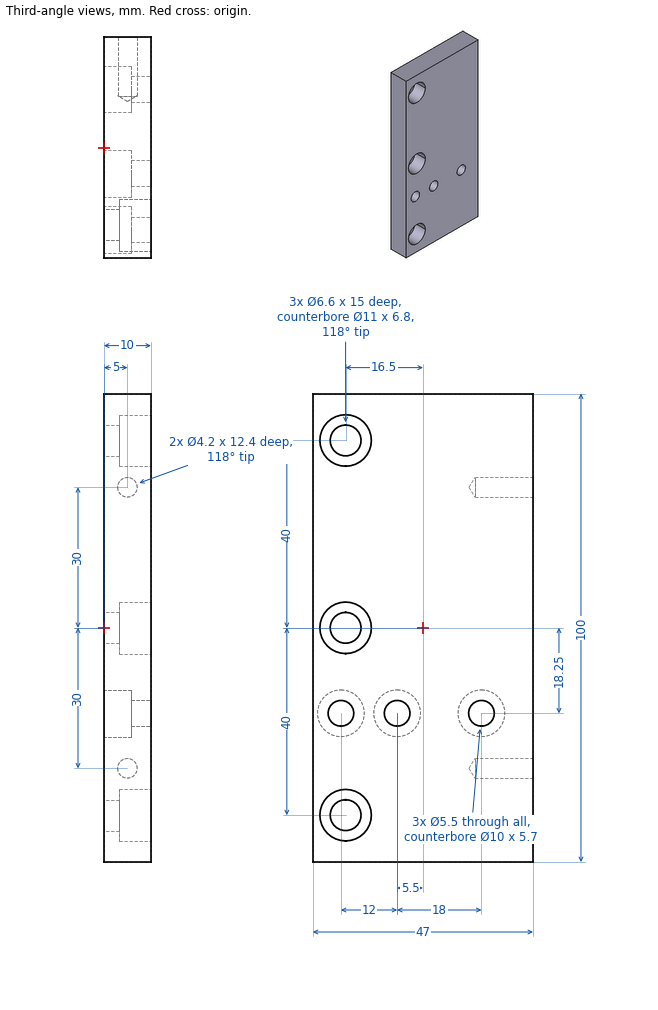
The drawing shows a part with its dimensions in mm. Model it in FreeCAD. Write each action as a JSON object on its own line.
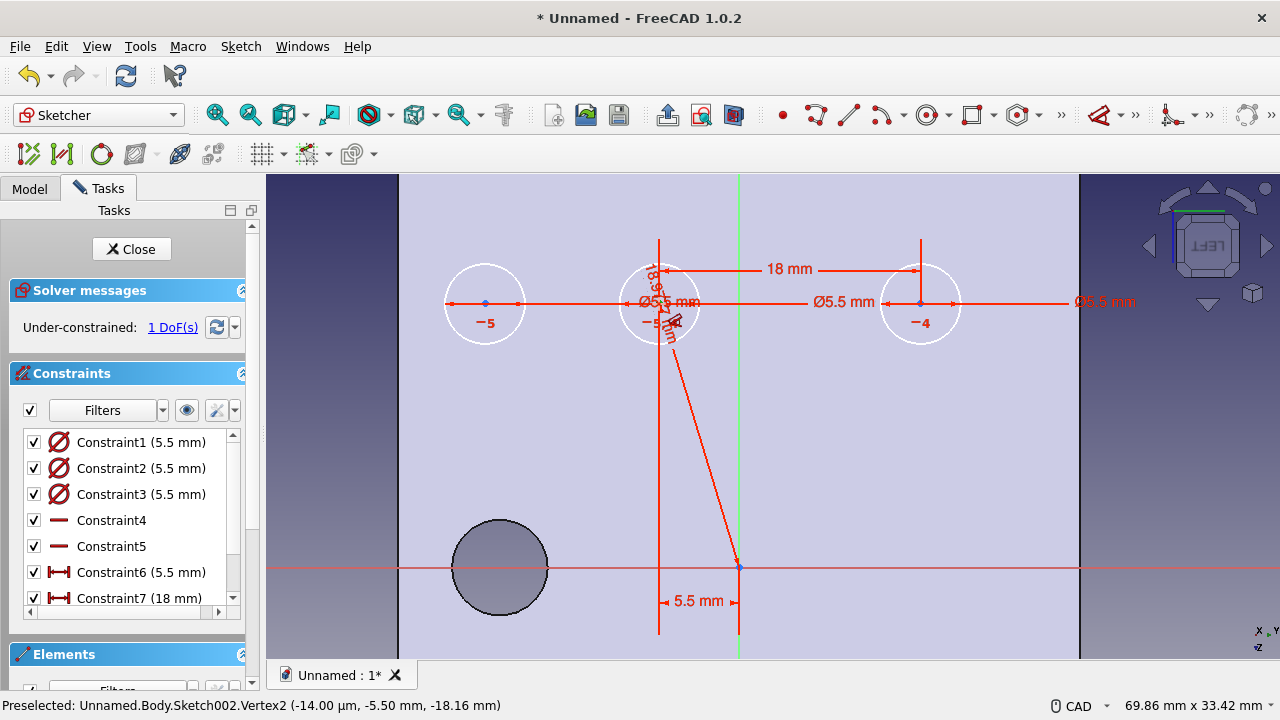
{"action": "left_click", "coordinate": [485, 304]}
{"action": "left_click", "coordinate": [572, 270]}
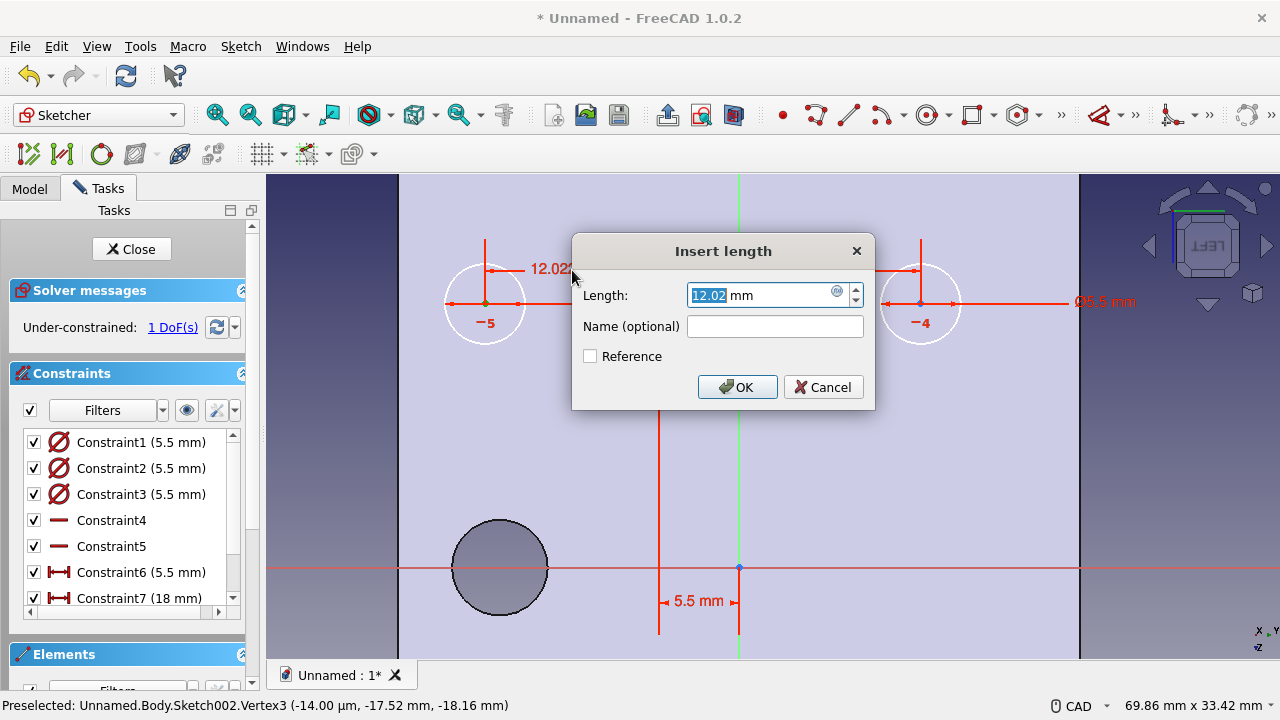
{"action": "type", "text": "12"}
{"action": "key", "text": "Return"}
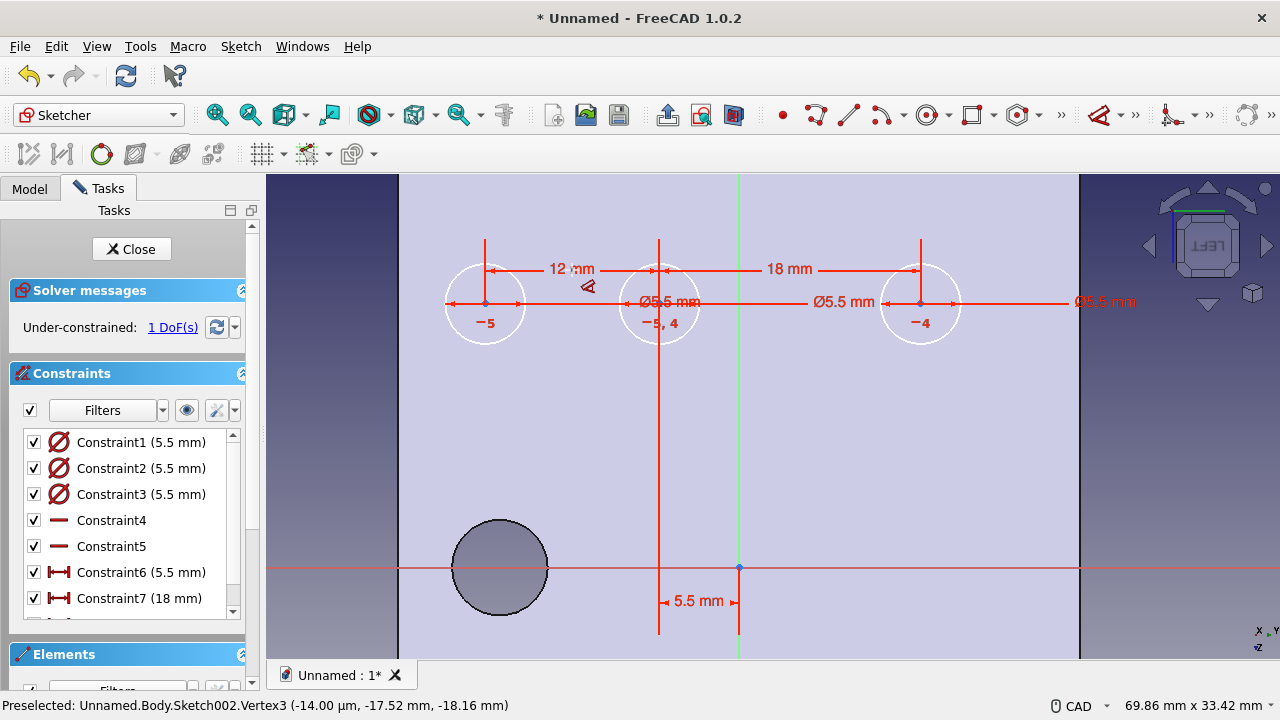
{"action": "left_click", "coordinate": [921, 304]}
{"action": "left_click", "coordinate": [955, 436]}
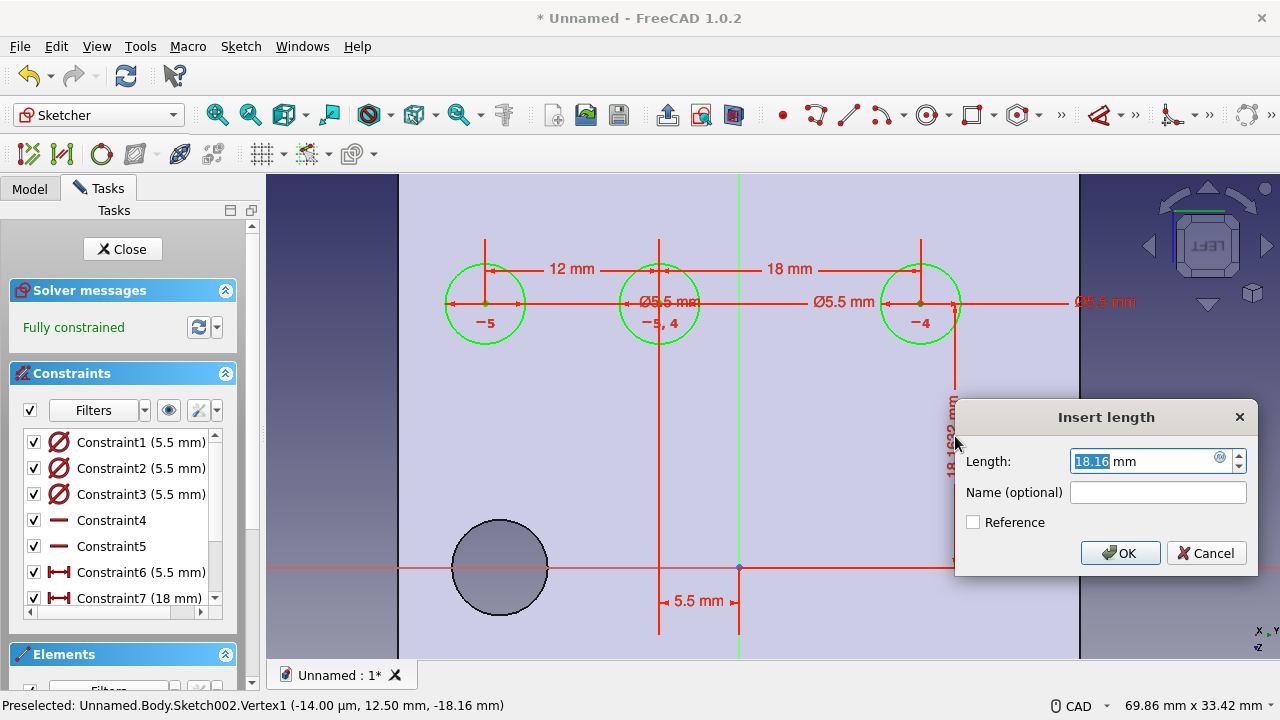
{"action": "type", "text": "18.25"}
{"action": "key", "text": "Return"}
{"action": "key", "text": "Escape"}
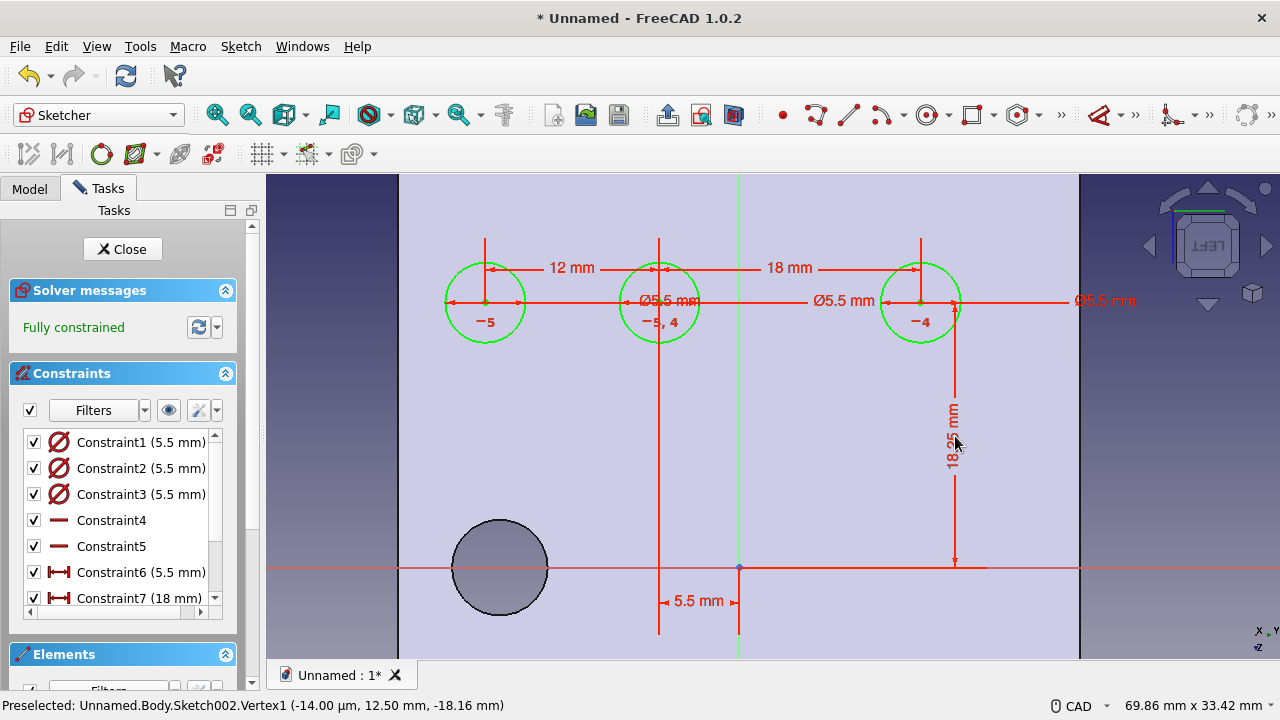
{"action": "left_click", "coordinate": [123, 249]}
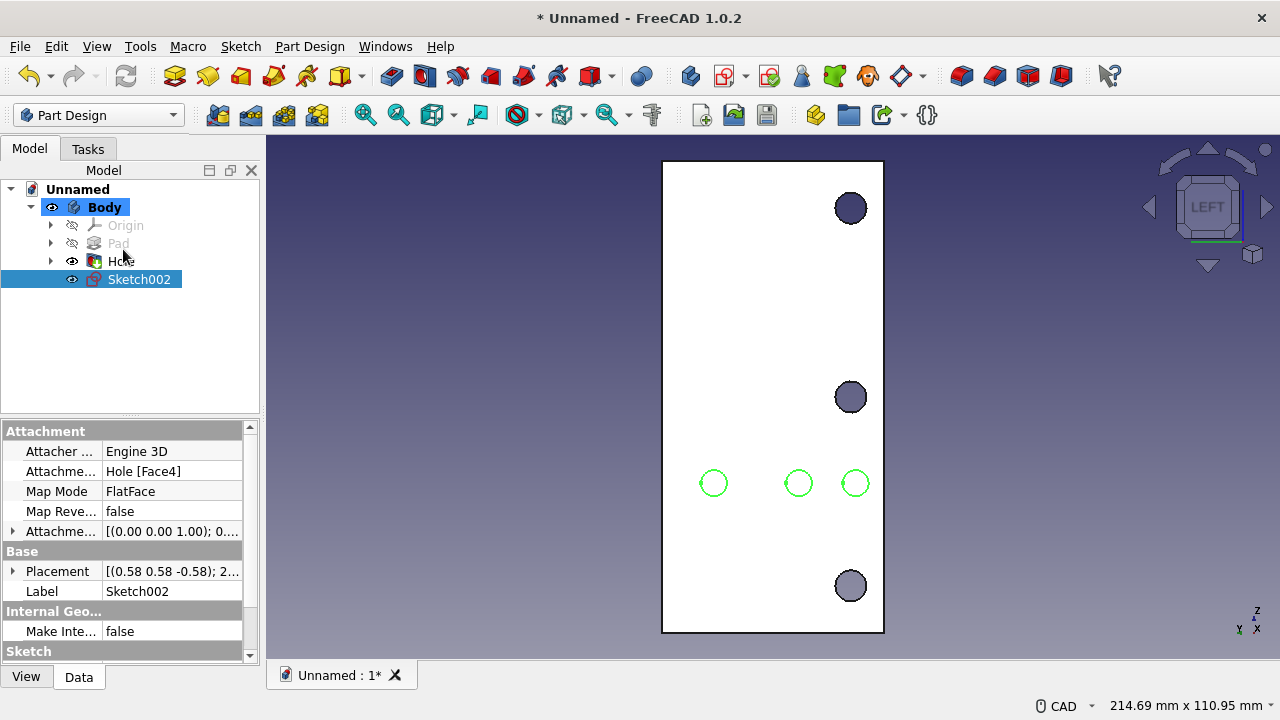
{"action": "left_click", "coordinate": [425, 76]}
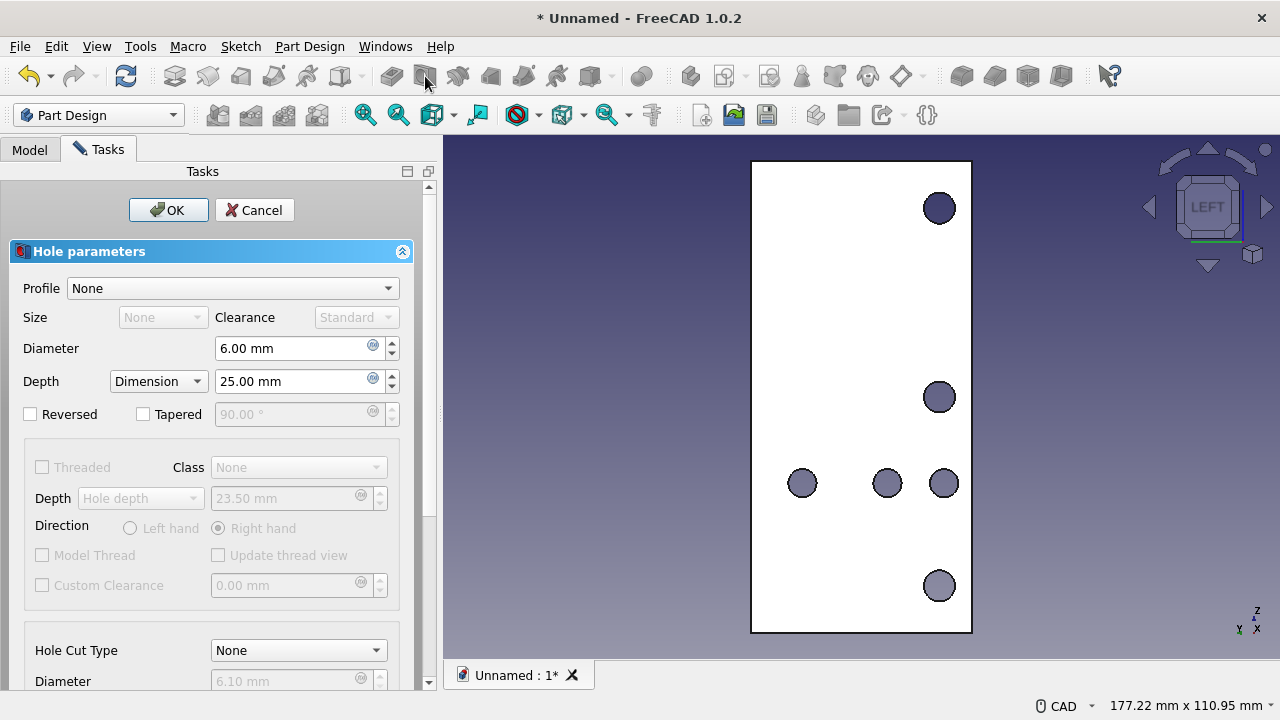
{"action": "triple_click", "coordinate": [300, 348]}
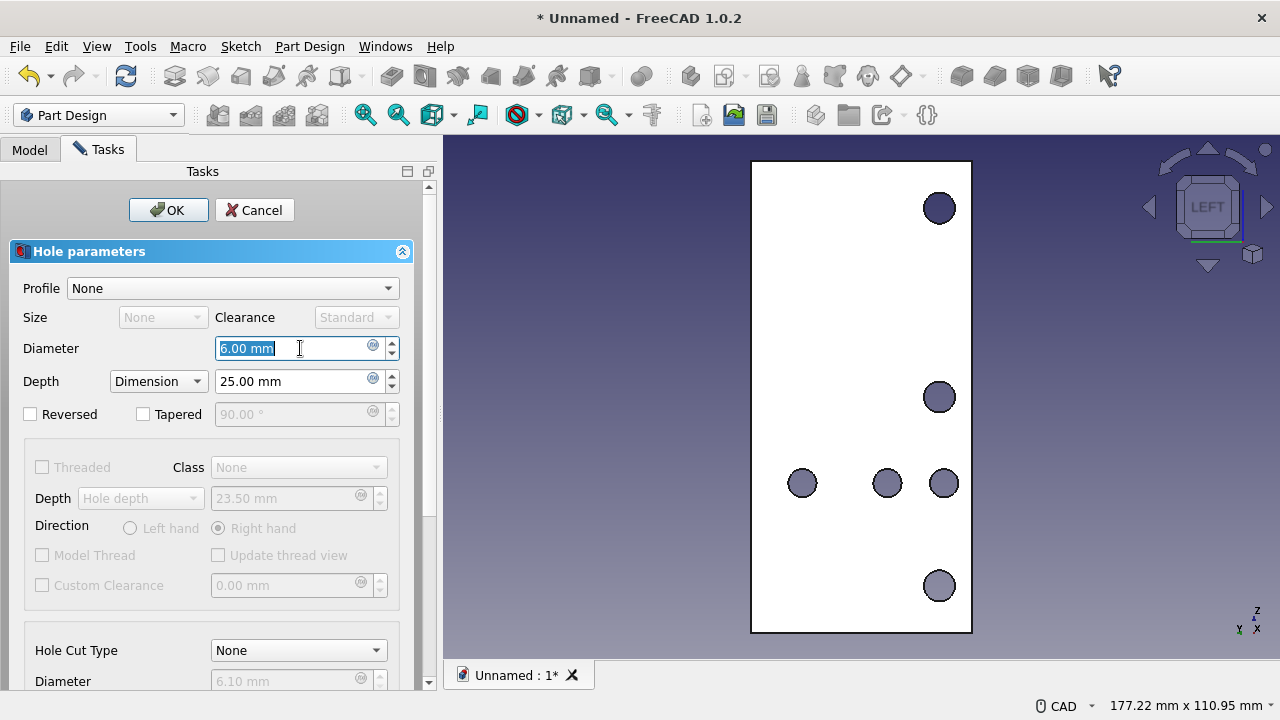
{"action": "type", "text": "5.5"}
{"action": "key", "text": "Tab"}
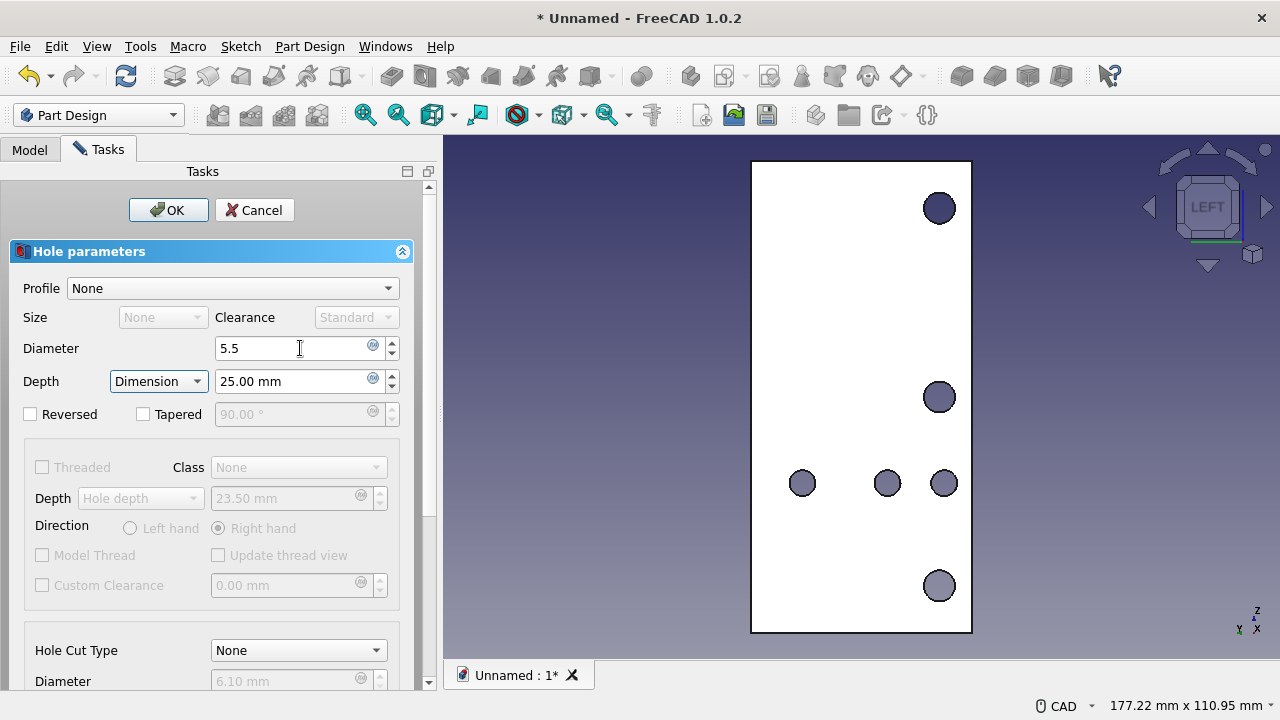
{"action": "left_click", "coordinate": [160, 382]}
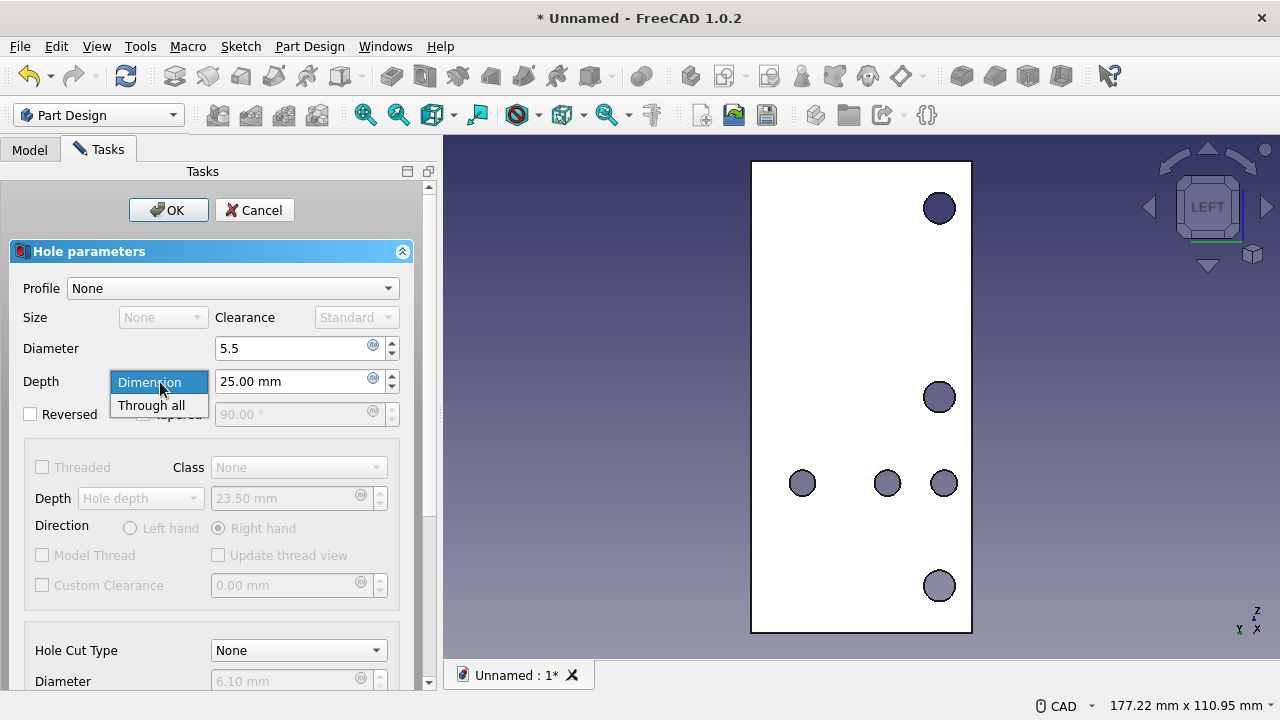
{"action": "left_click", "coordinate": [158, 406]}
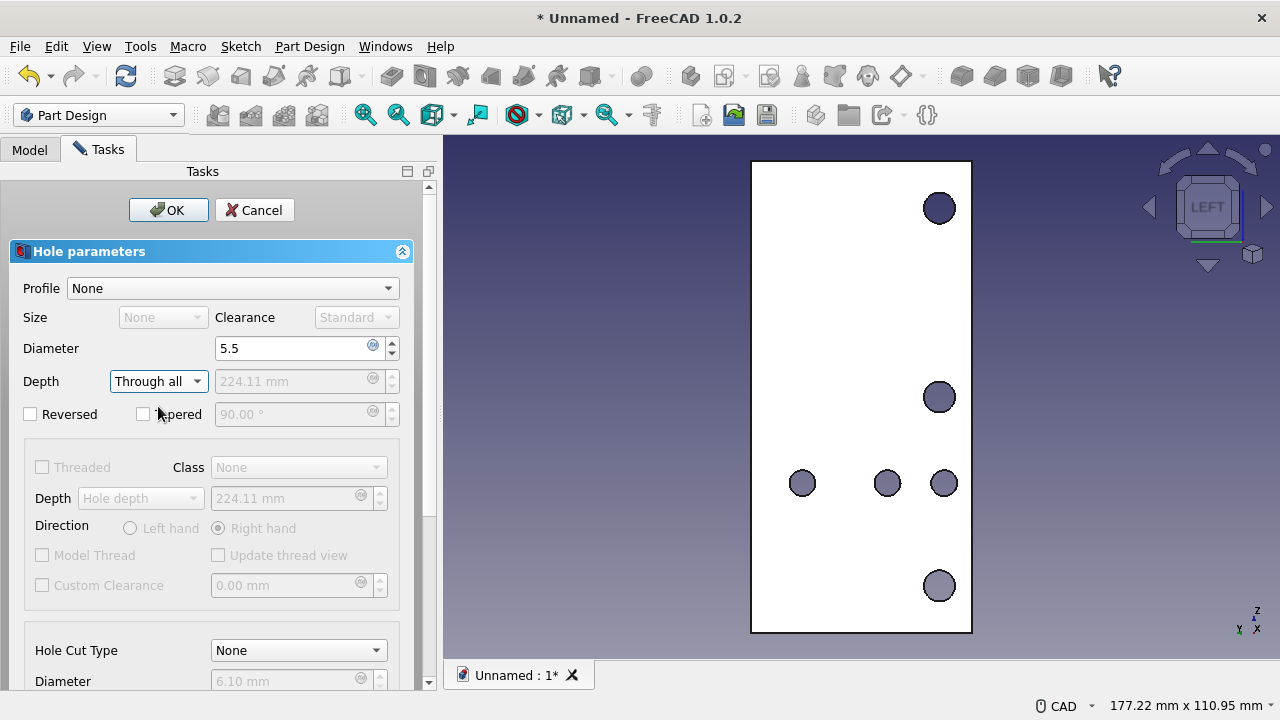
{"action": "left_click", "coordinate": [300, 650]}